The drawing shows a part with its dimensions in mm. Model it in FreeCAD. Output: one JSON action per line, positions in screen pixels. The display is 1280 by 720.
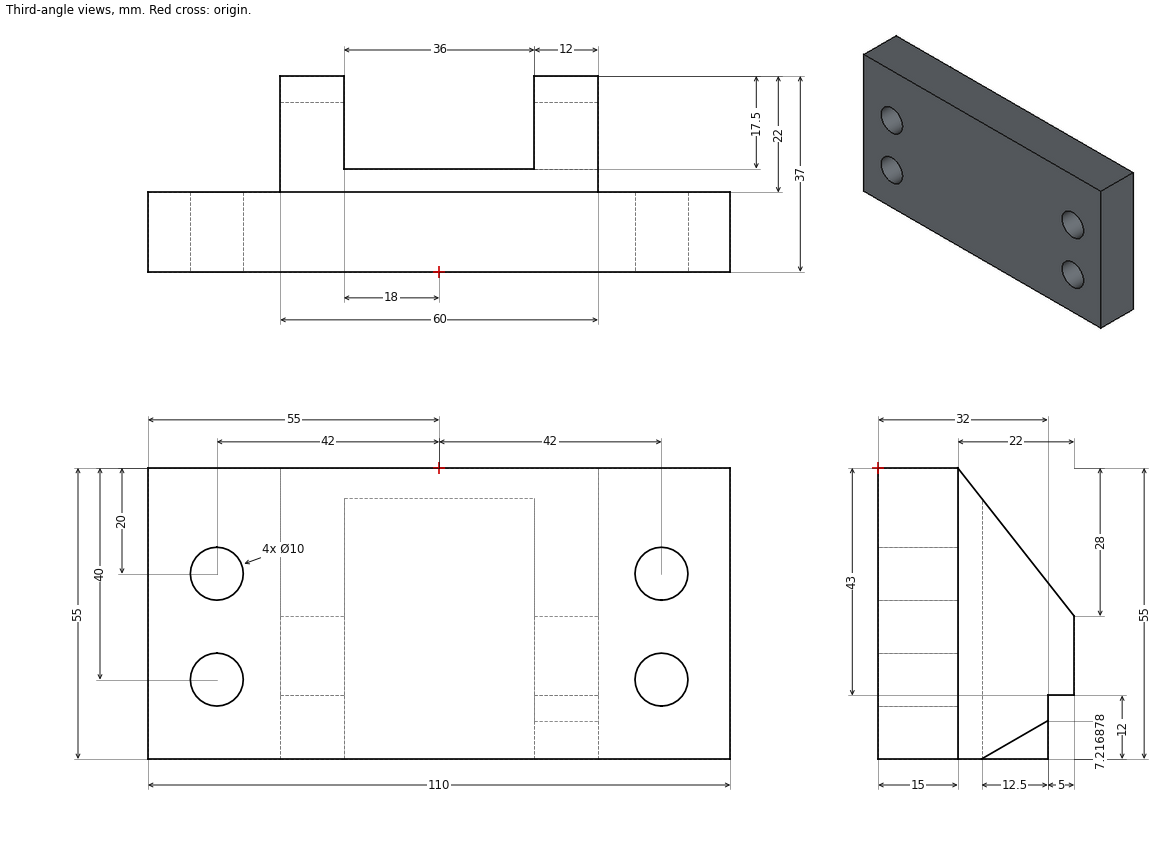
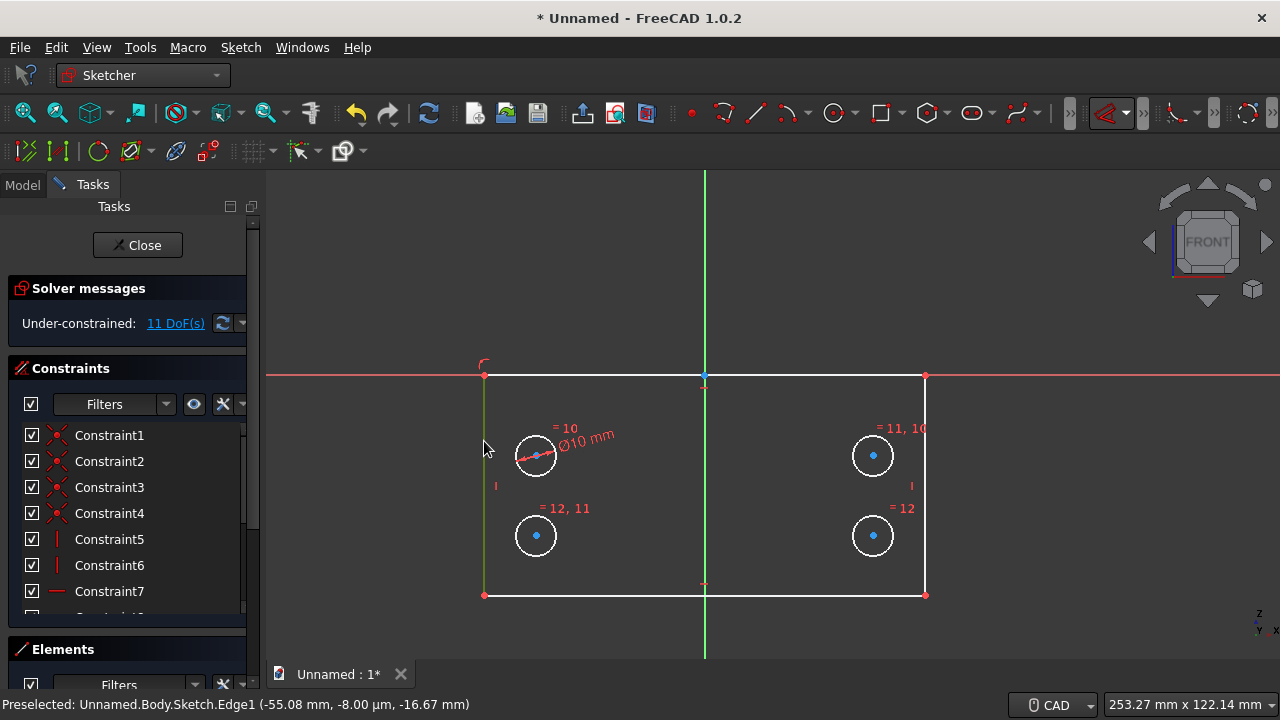
{"action": "left_click", "coordinate": [1128, 114]}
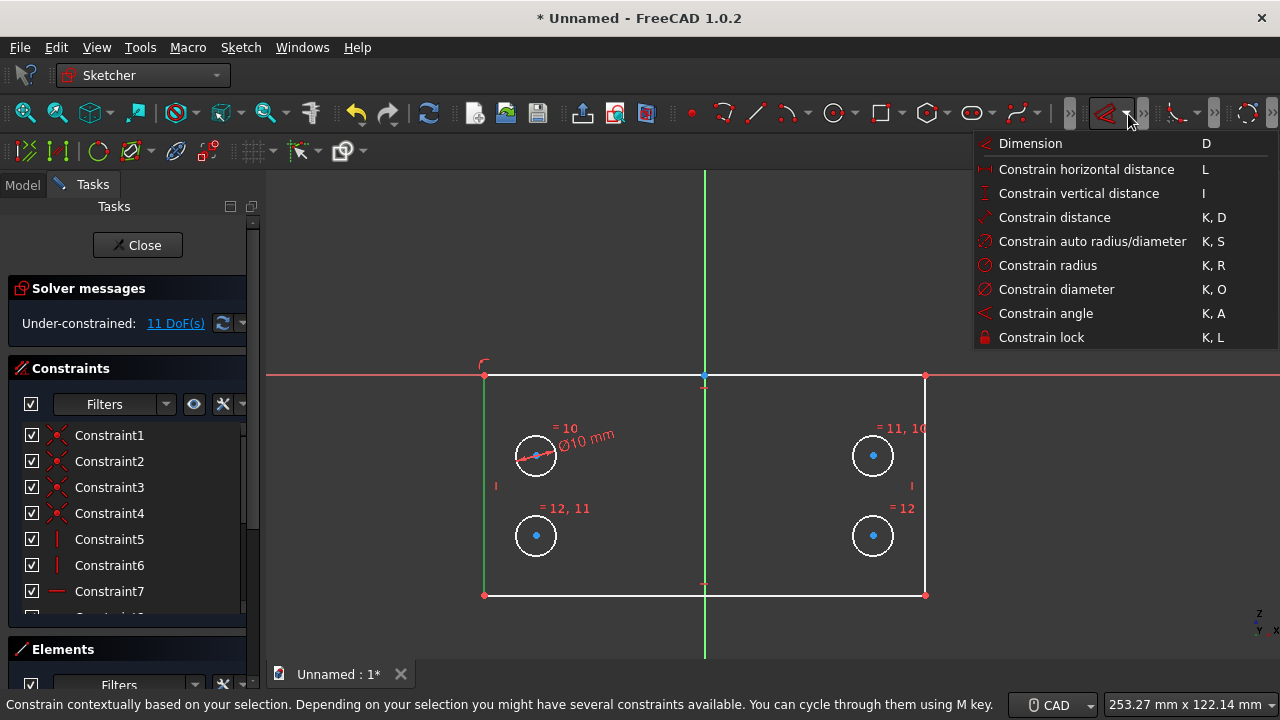
{"action": "left_click", "coordinate": [1126, 193]}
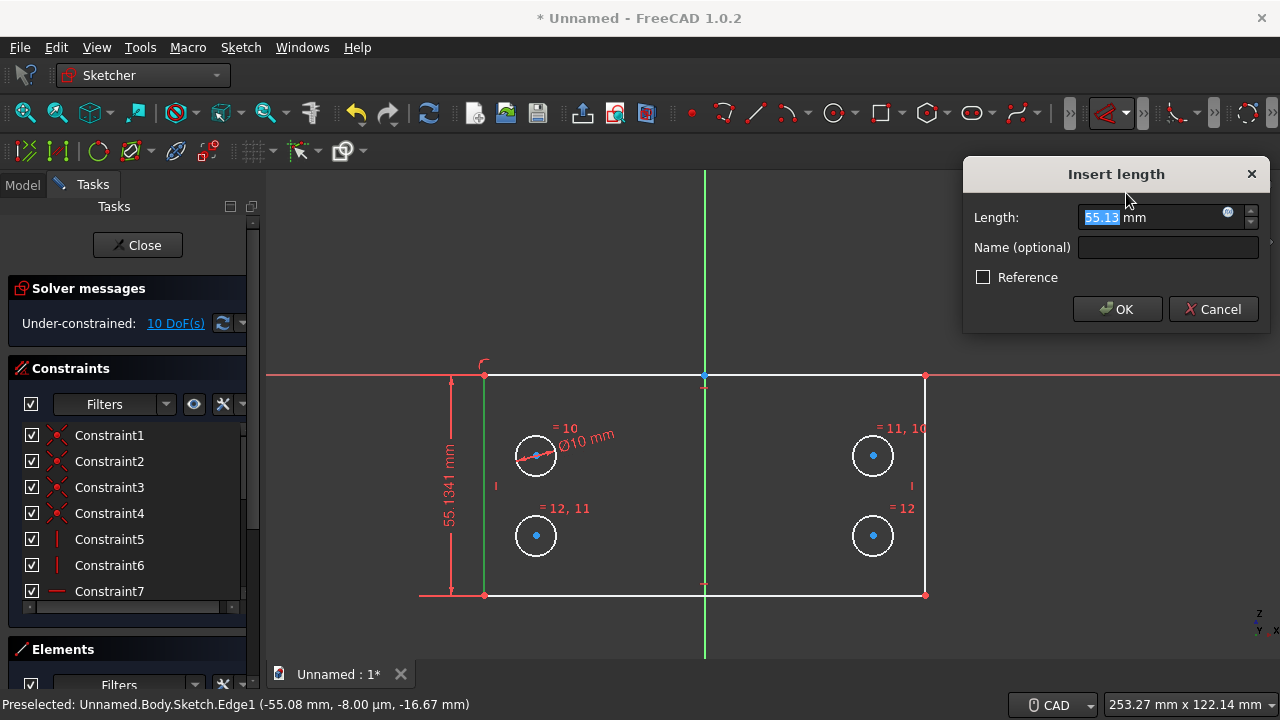
{"action": "type", "text": "55"}
{"action": "key", "text": "Return"}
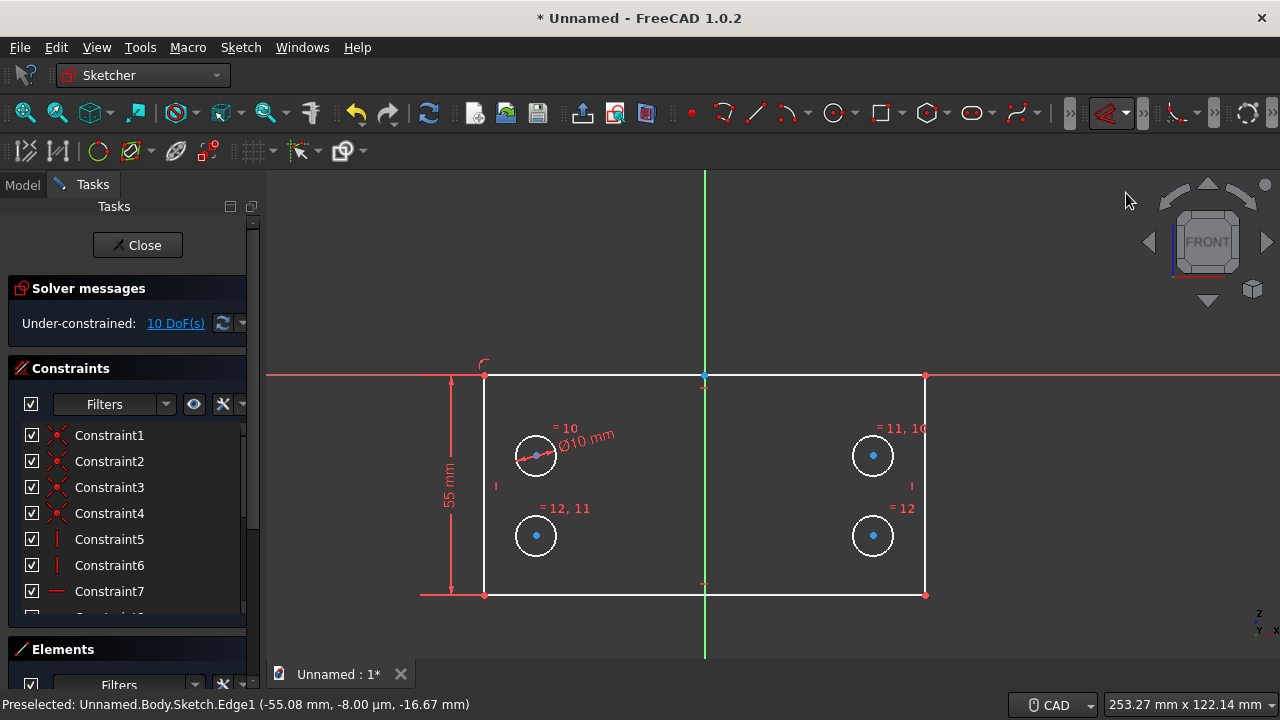
{"action": "left_click", "coordinate": [536, 456]}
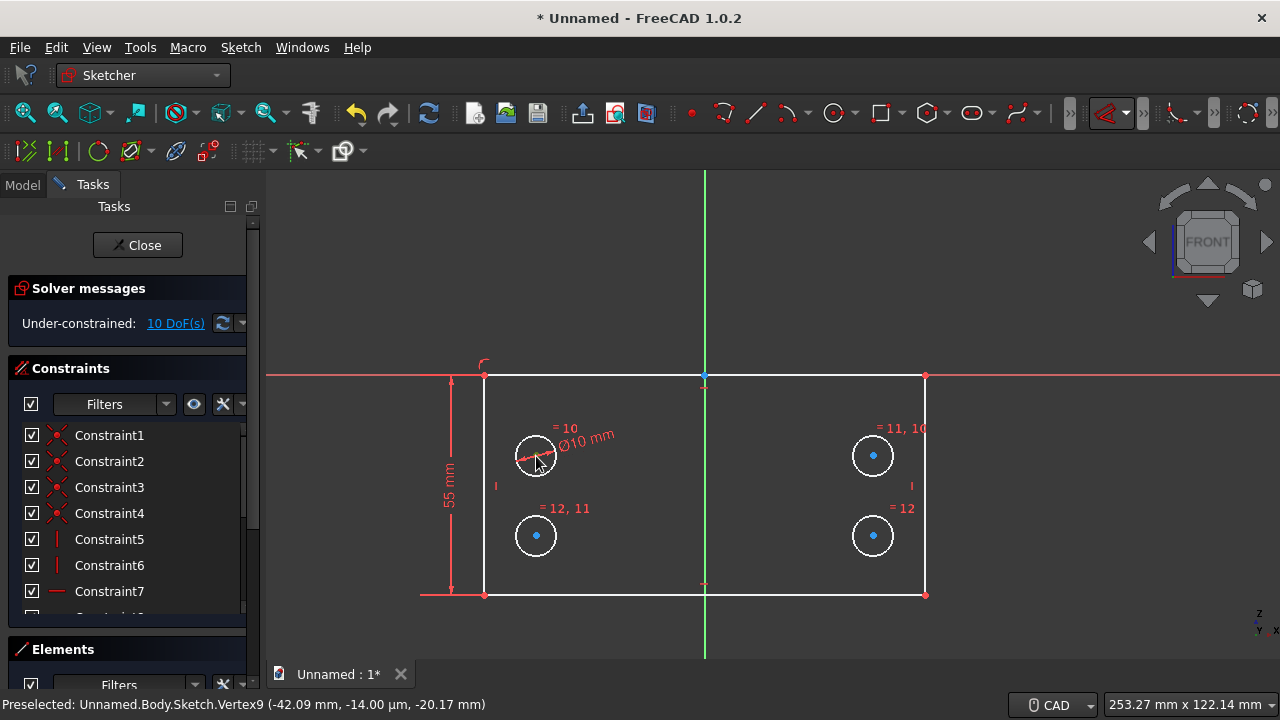
{"action": "key", "text": "l"}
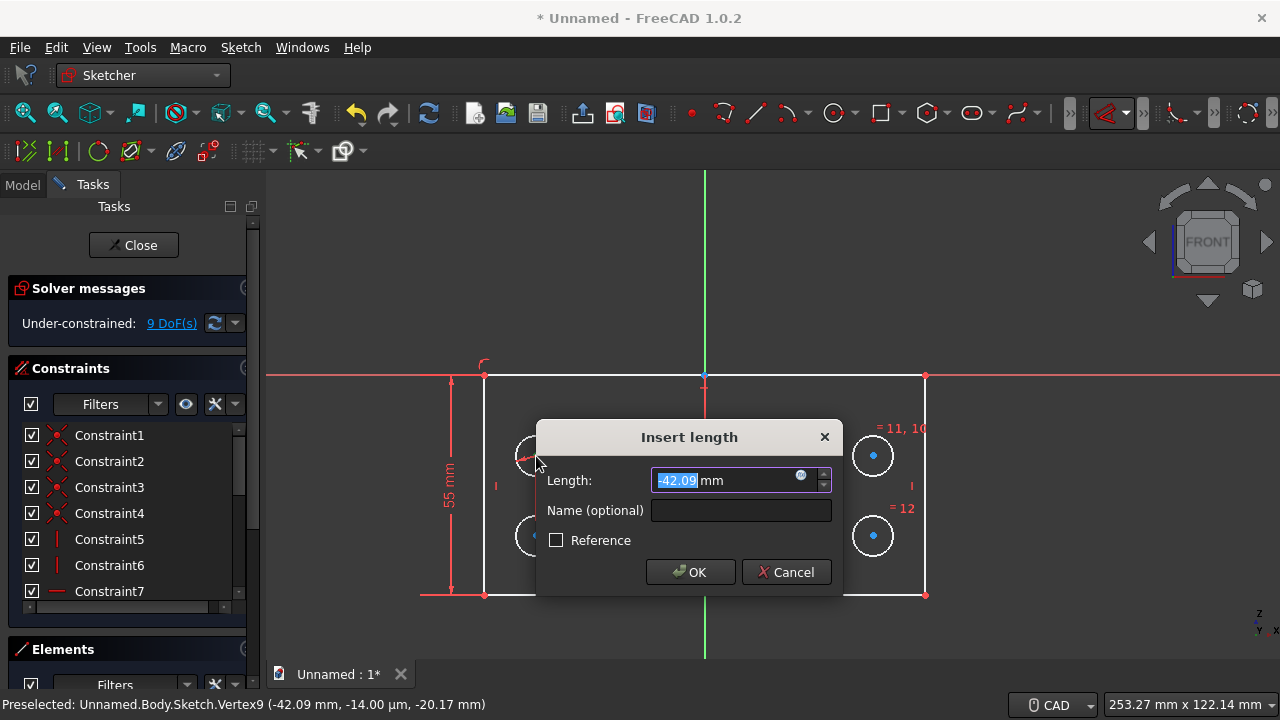
{"action": "type", "text": "-42"}
{"action": "key", "text": "Return"}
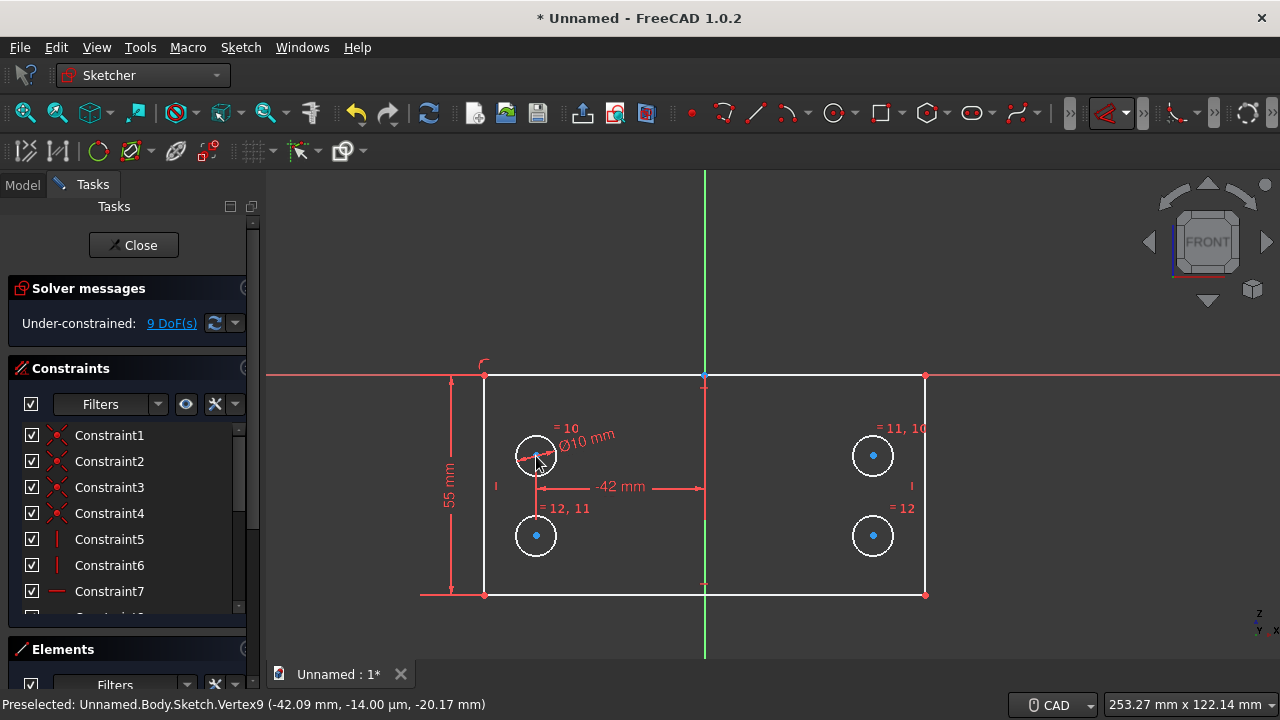
{"action": "left_click", "coordinate": [536, 456]}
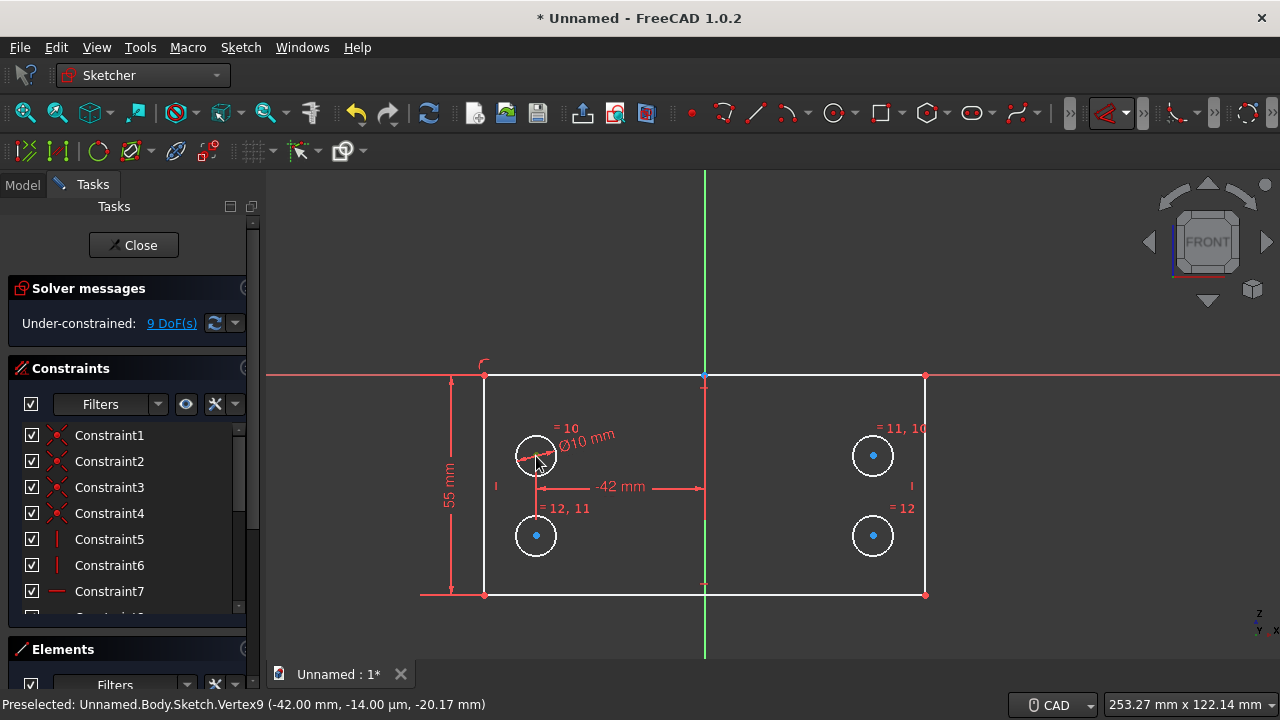
{"action": "key", "text": "i"}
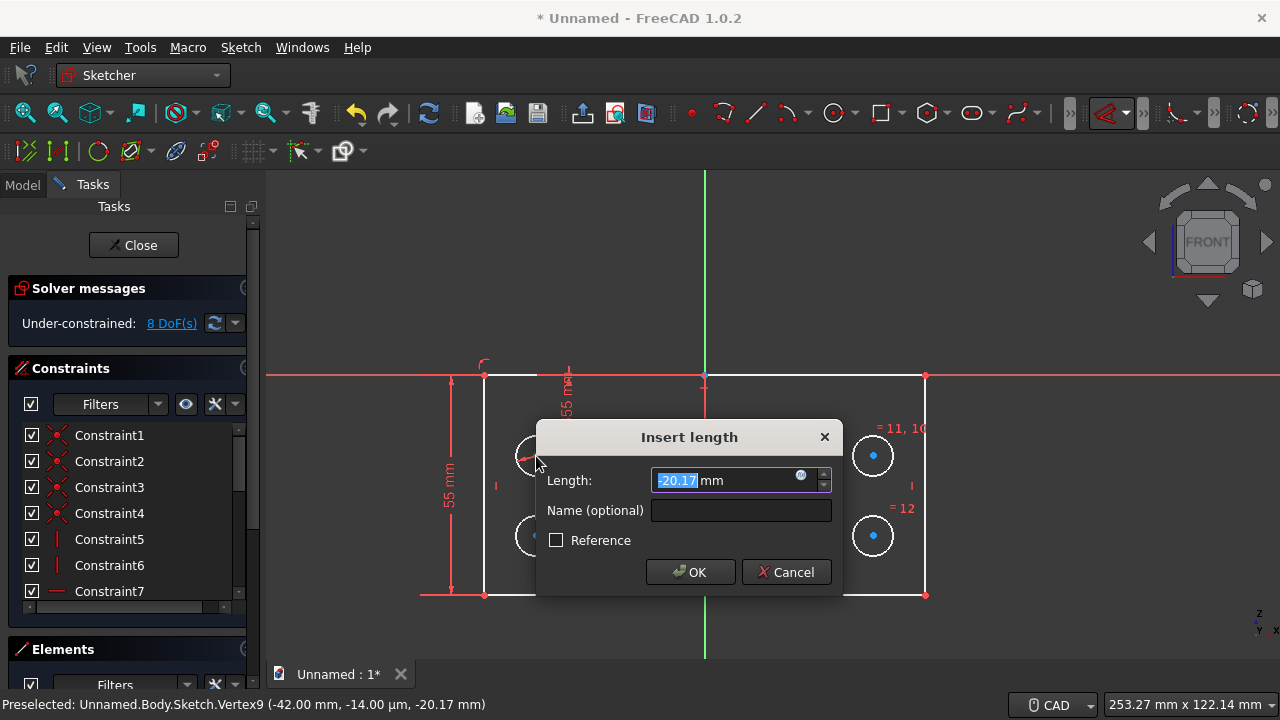
{"action": "type", "text": "-20"}
{"action": "key", "text": "Return"}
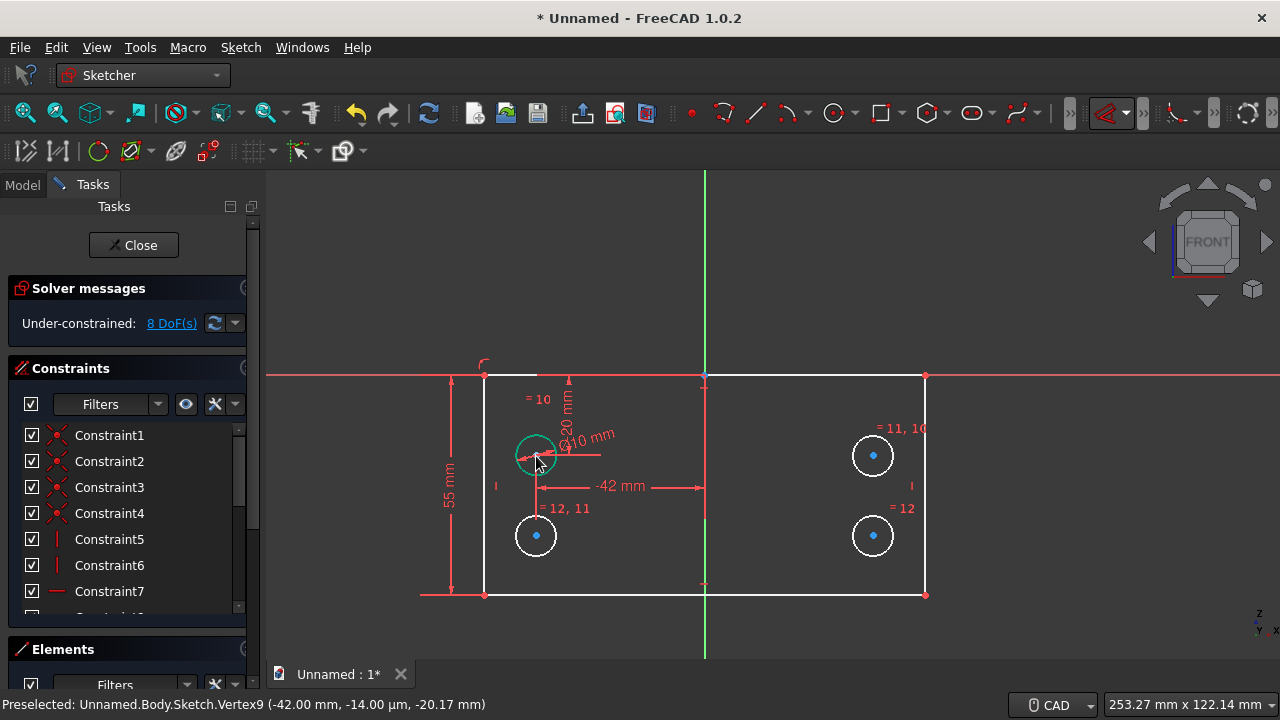
{"action": "left_click", "coordinate": [873, 456]}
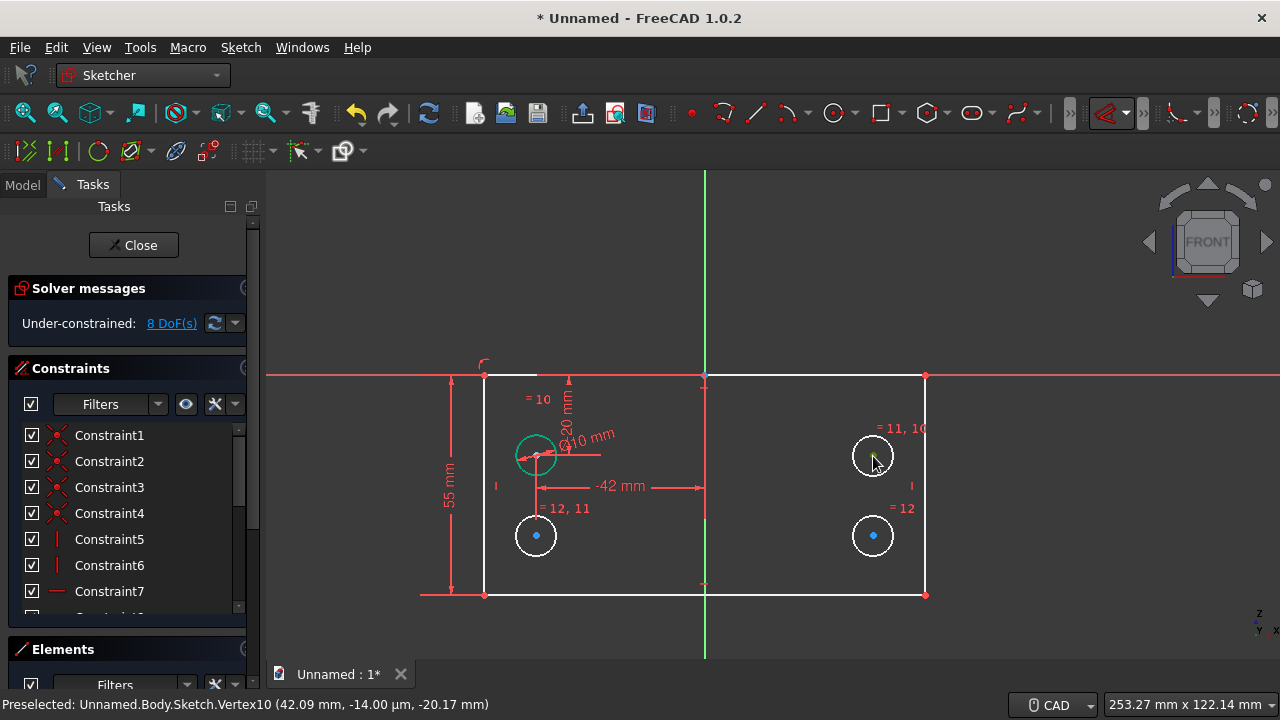
{"action": "key", "text": "l"}